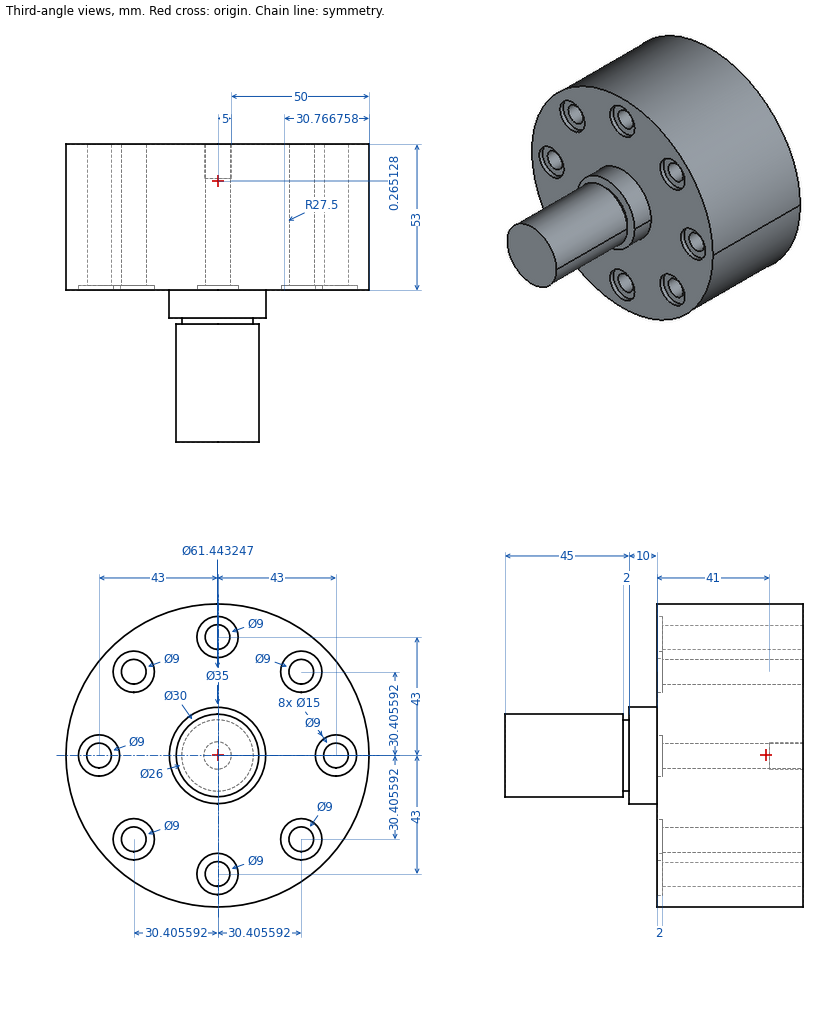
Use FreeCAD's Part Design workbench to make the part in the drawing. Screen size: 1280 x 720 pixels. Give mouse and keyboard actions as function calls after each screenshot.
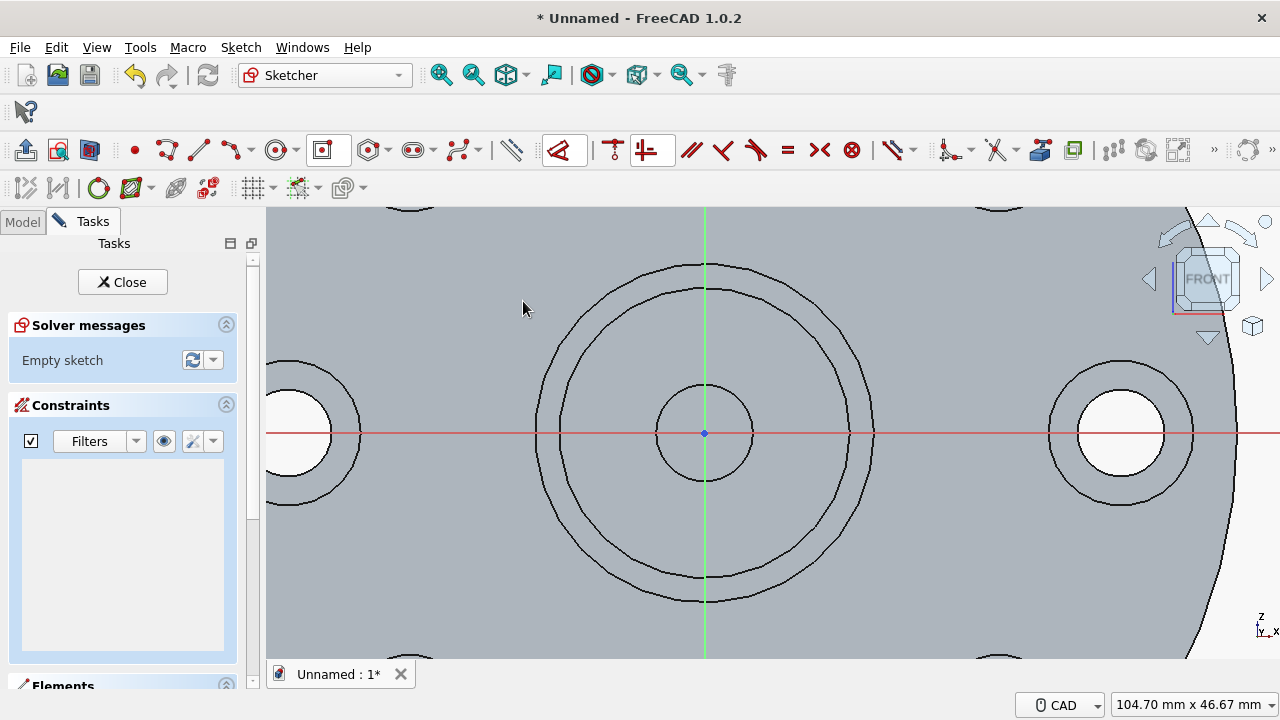
click(276, 150)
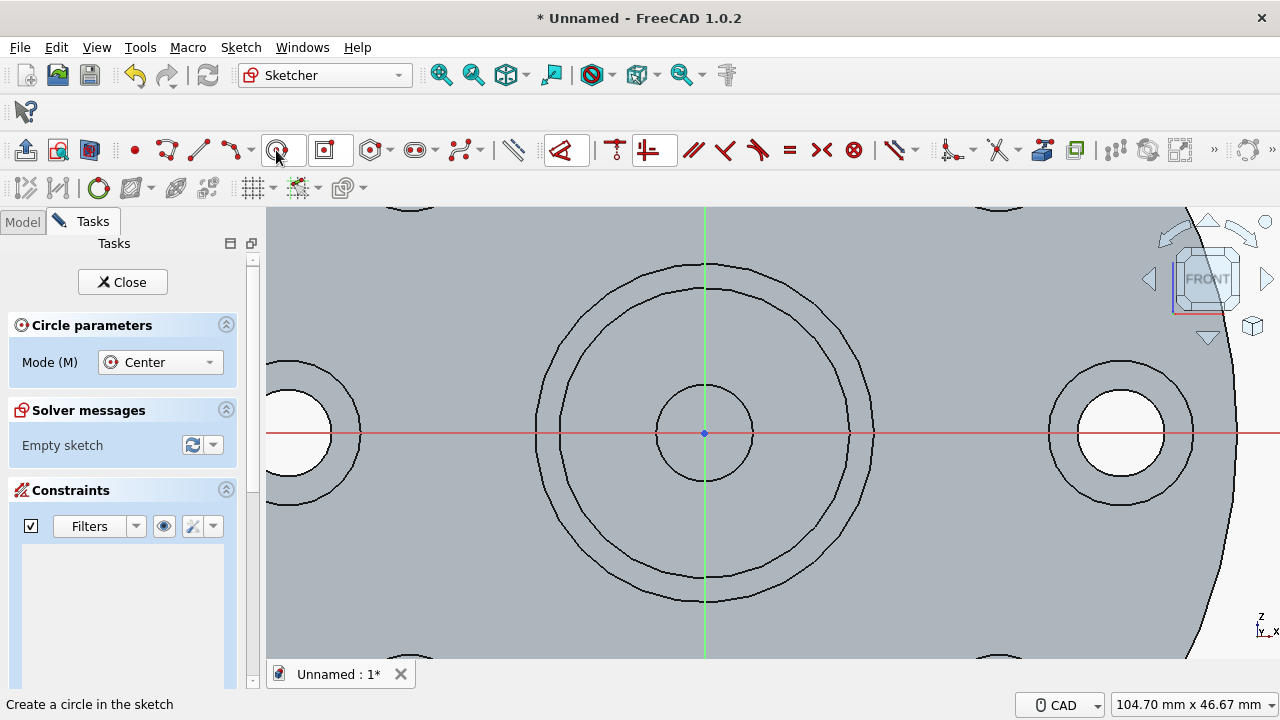
click(705, 433)
move(807, 330)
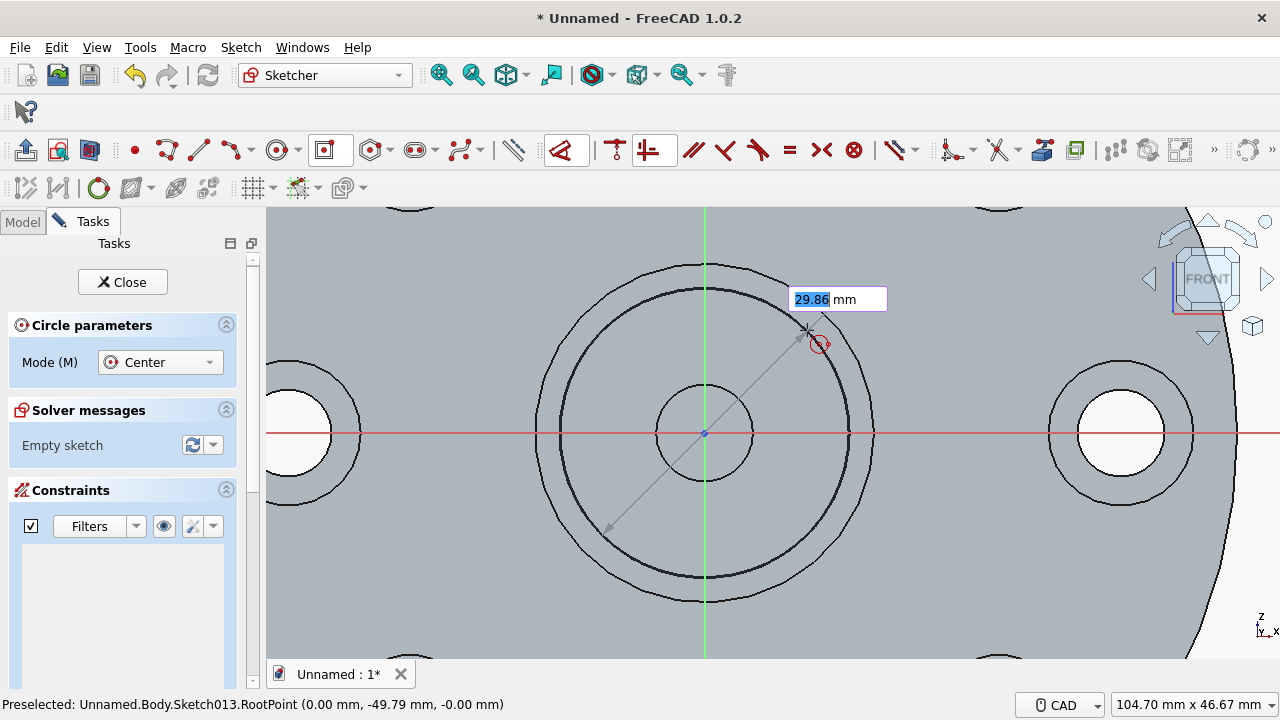
text(30)
key(Return)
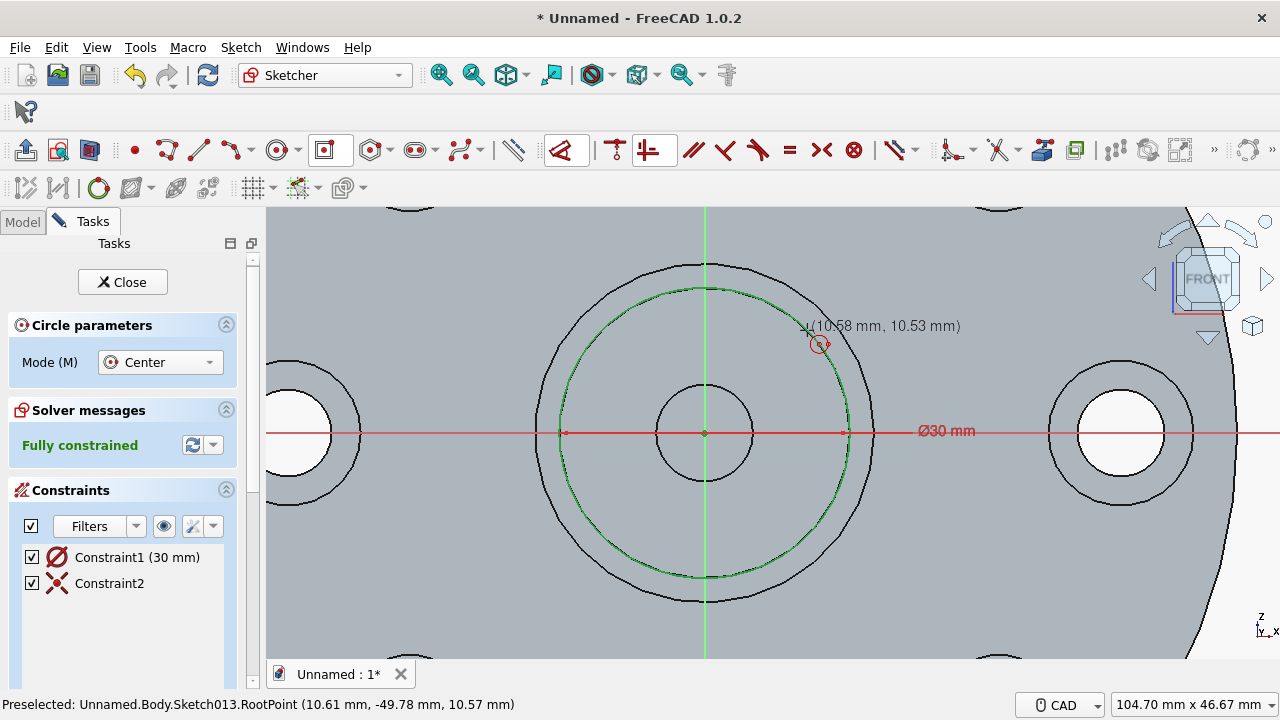
click(705, 433)
move(794, 344)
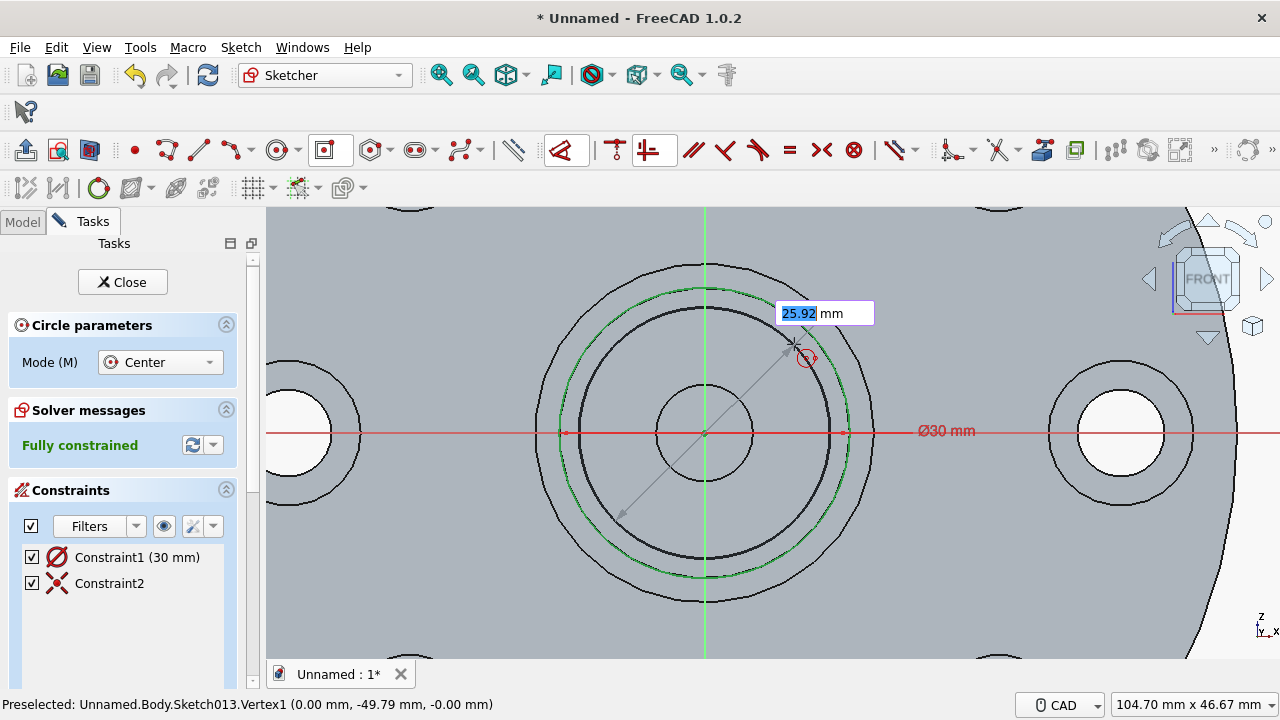
text(26)
key(Return)
key(Escape)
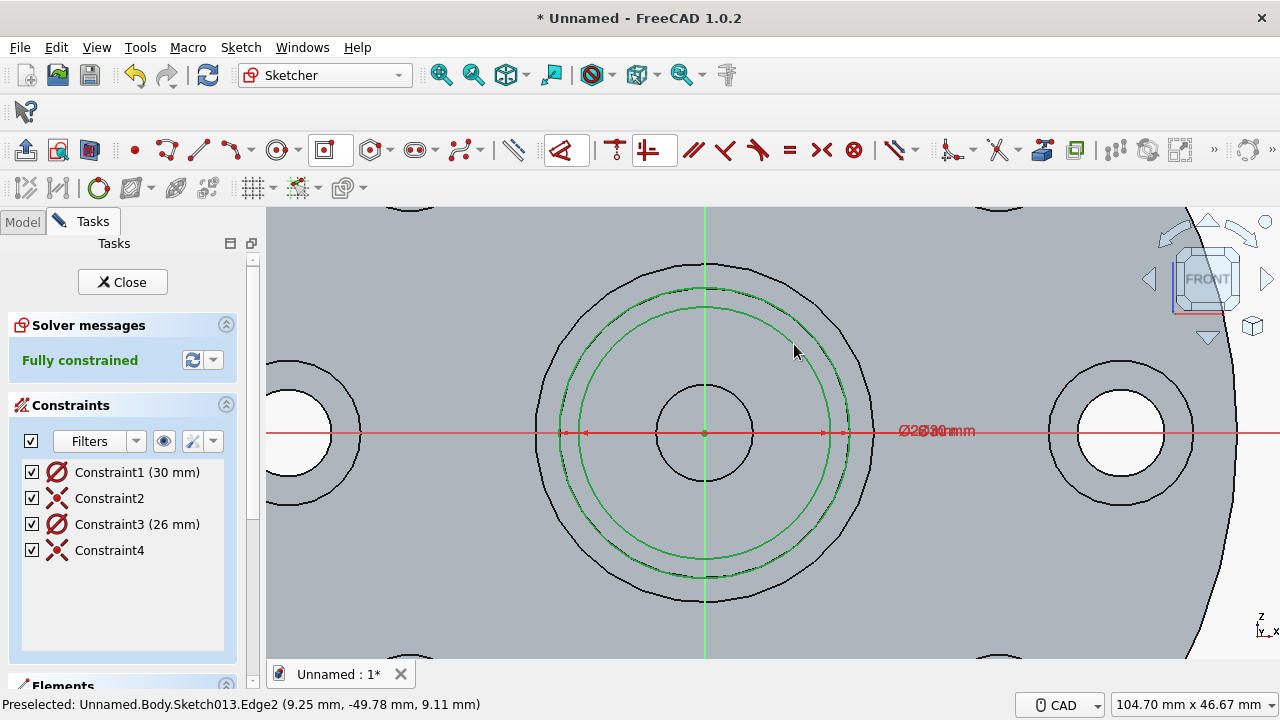
click(123, 282)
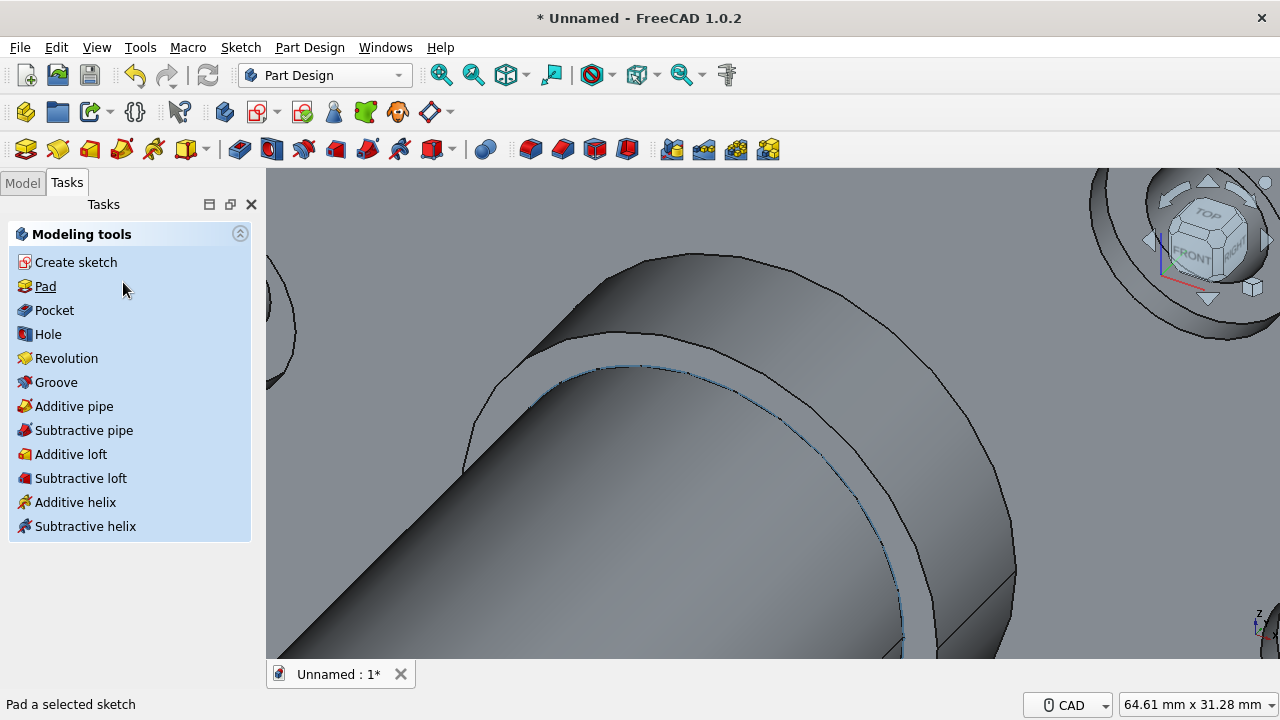
click(240, 150)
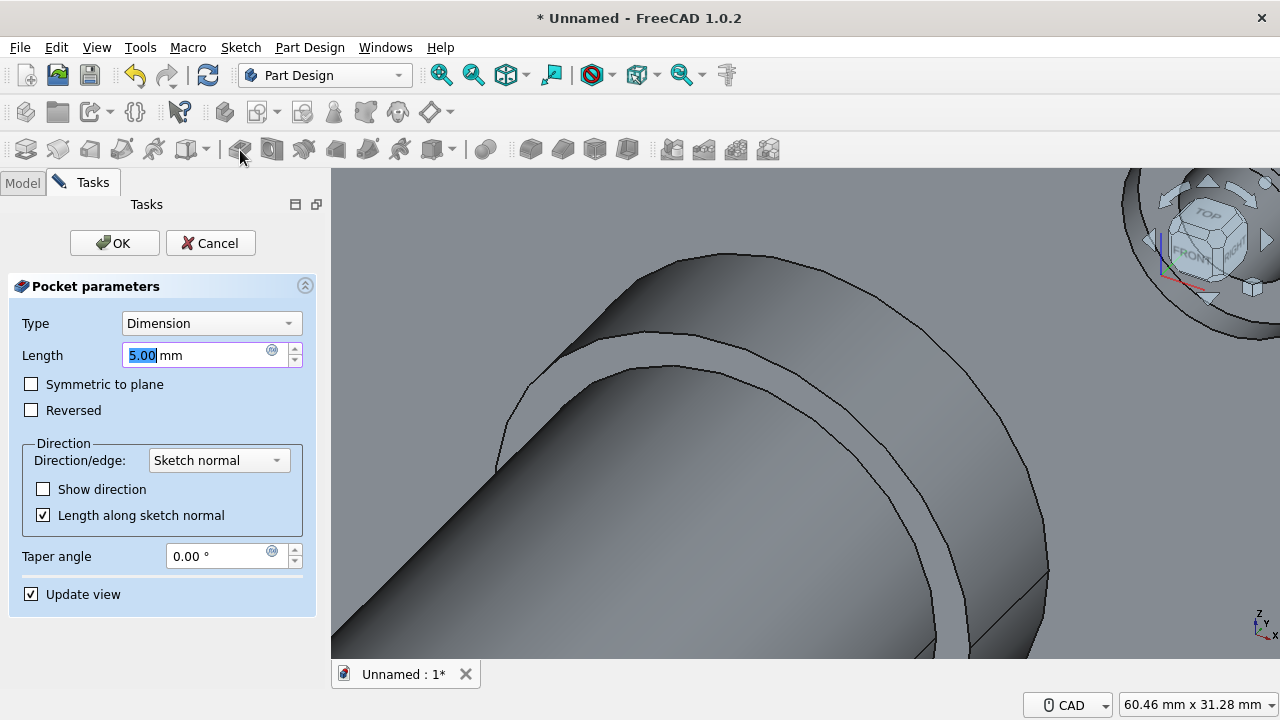
text(2)
key(Tab)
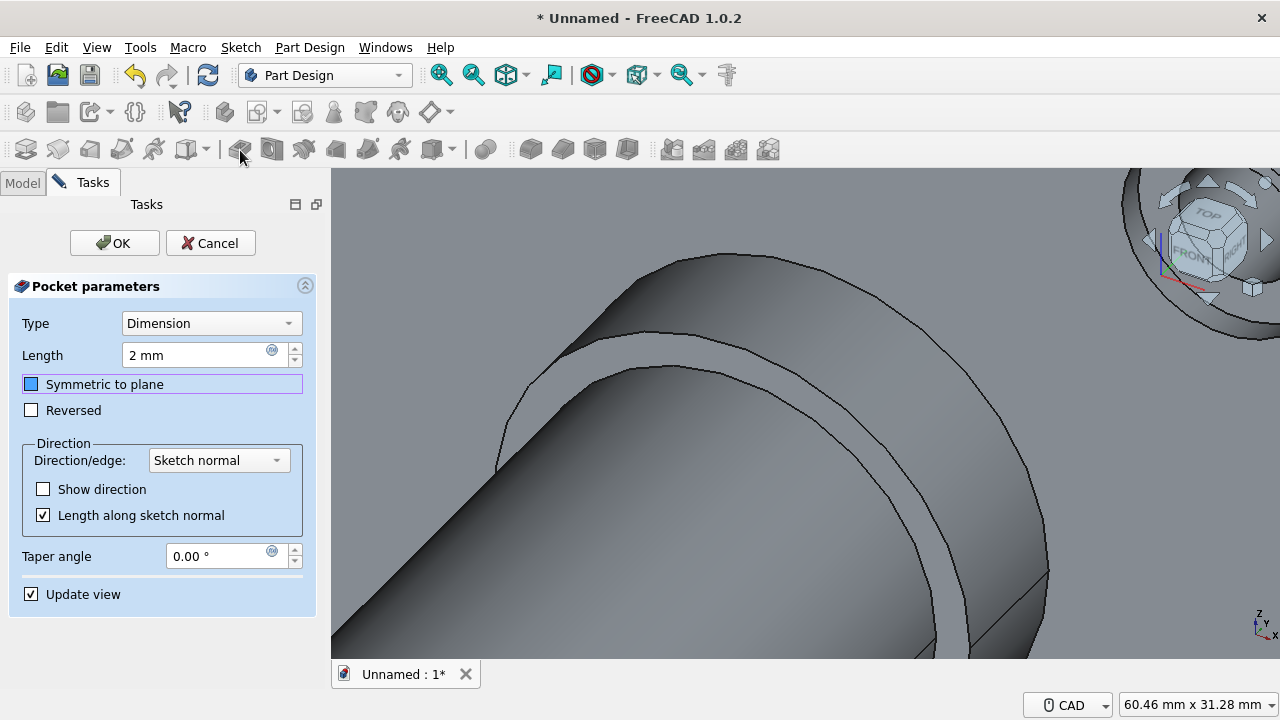
click(30, 410)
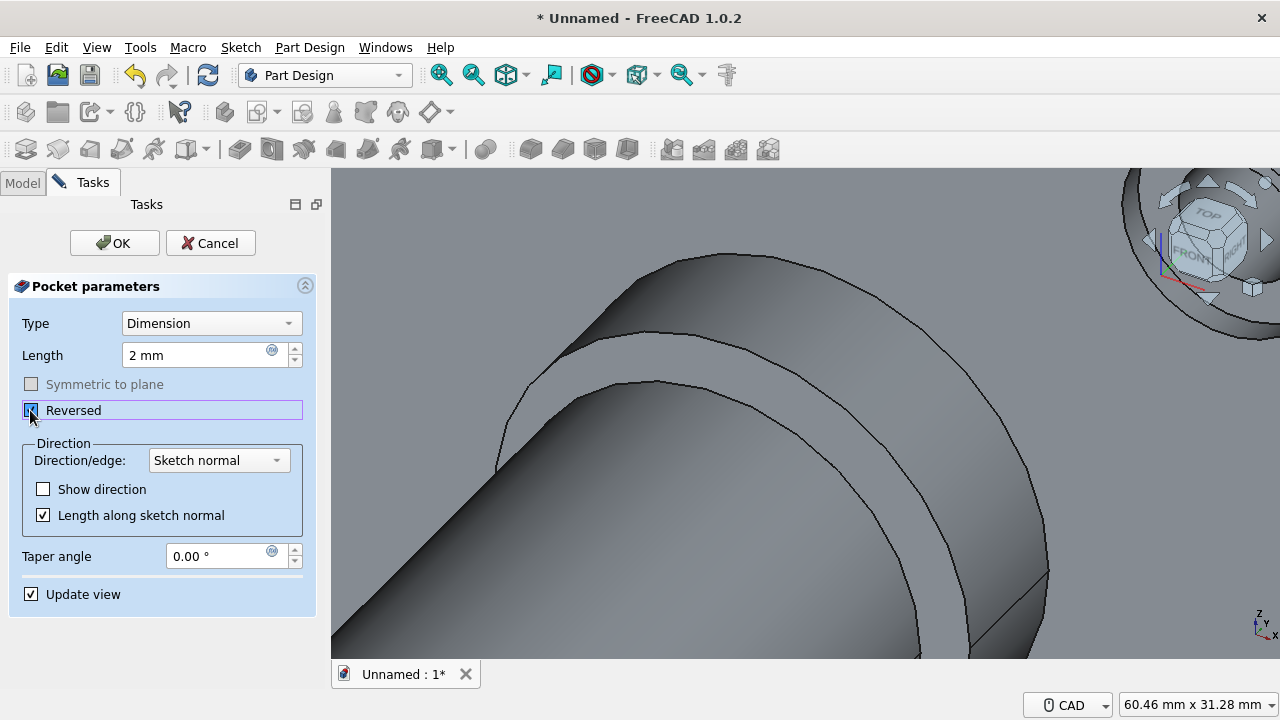
click(115, 243)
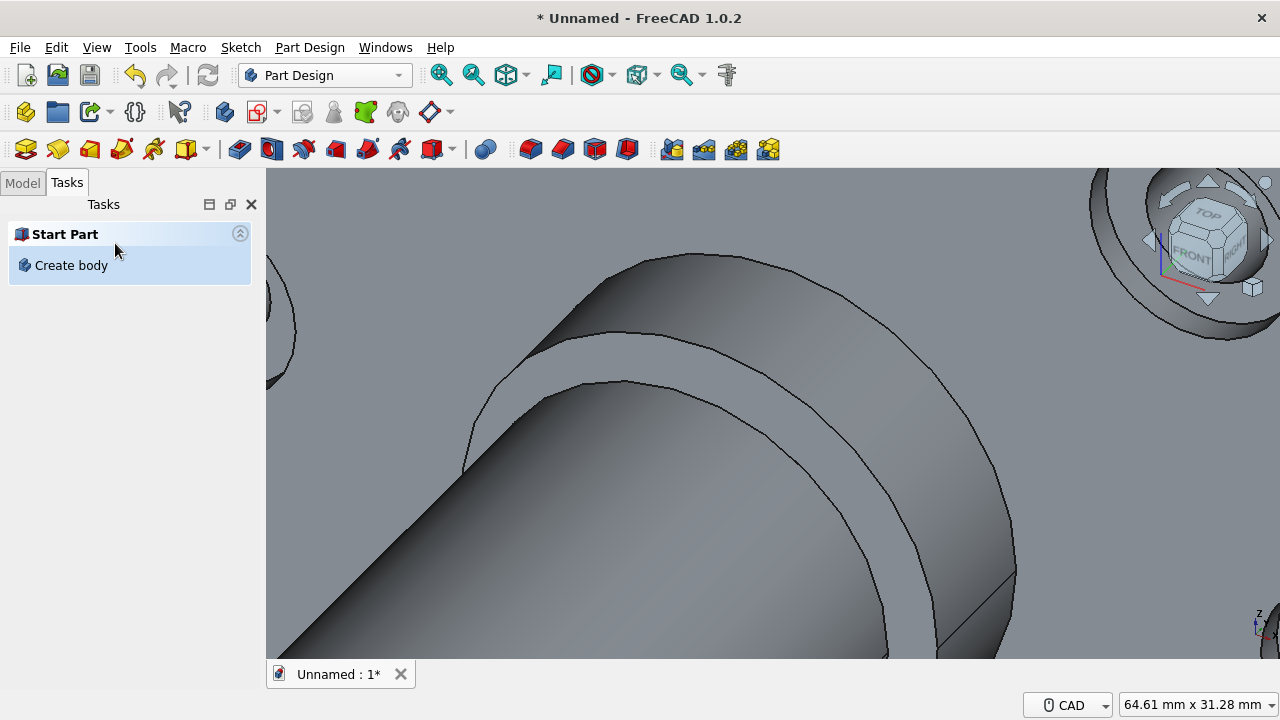
key(0)